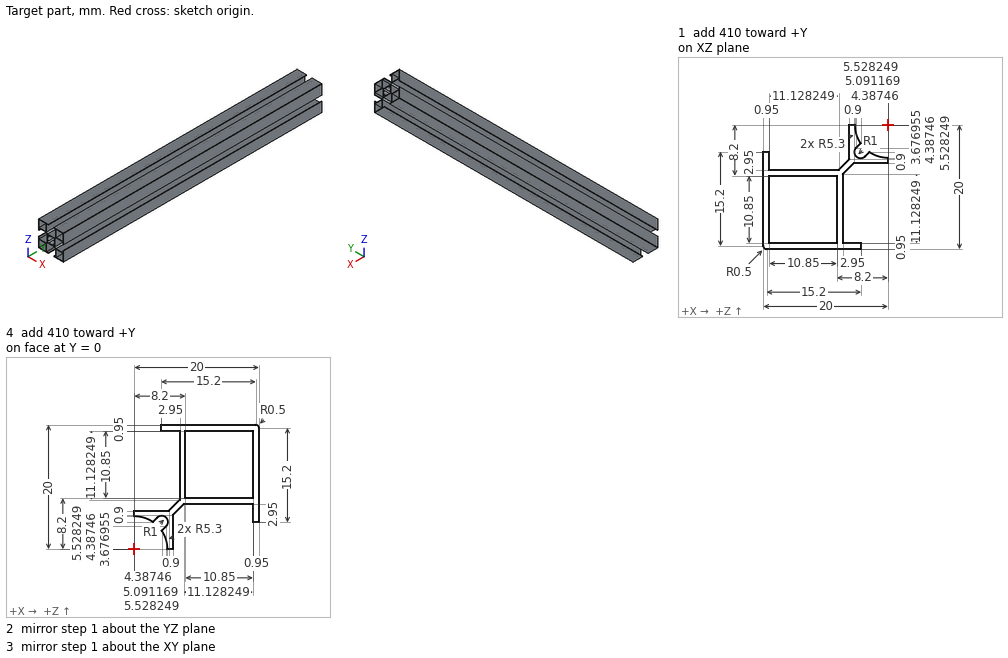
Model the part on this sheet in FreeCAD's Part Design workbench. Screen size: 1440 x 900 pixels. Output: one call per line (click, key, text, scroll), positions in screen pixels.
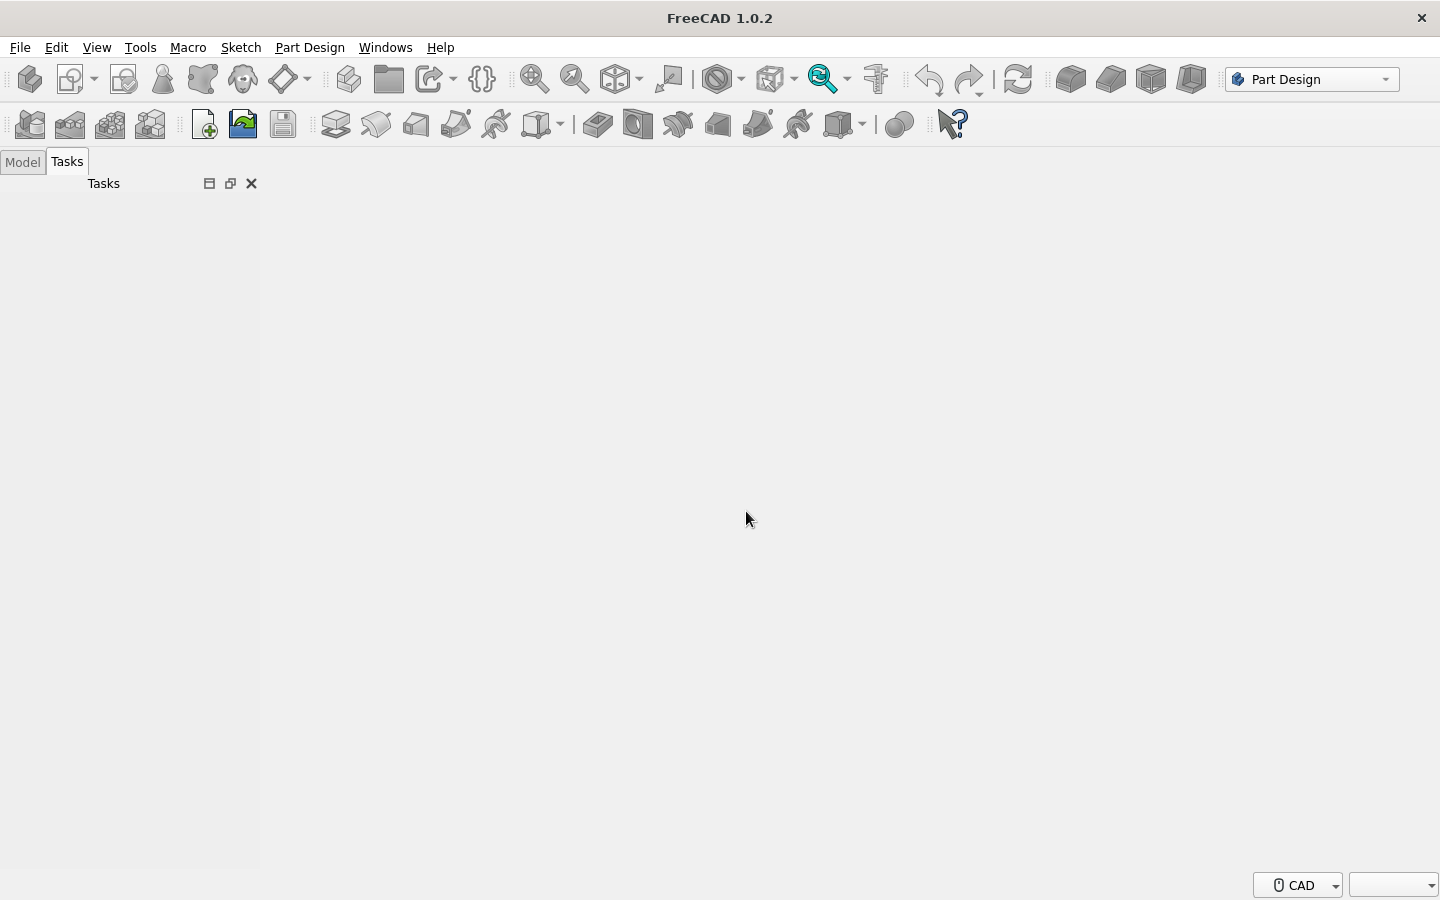
click(204, 124)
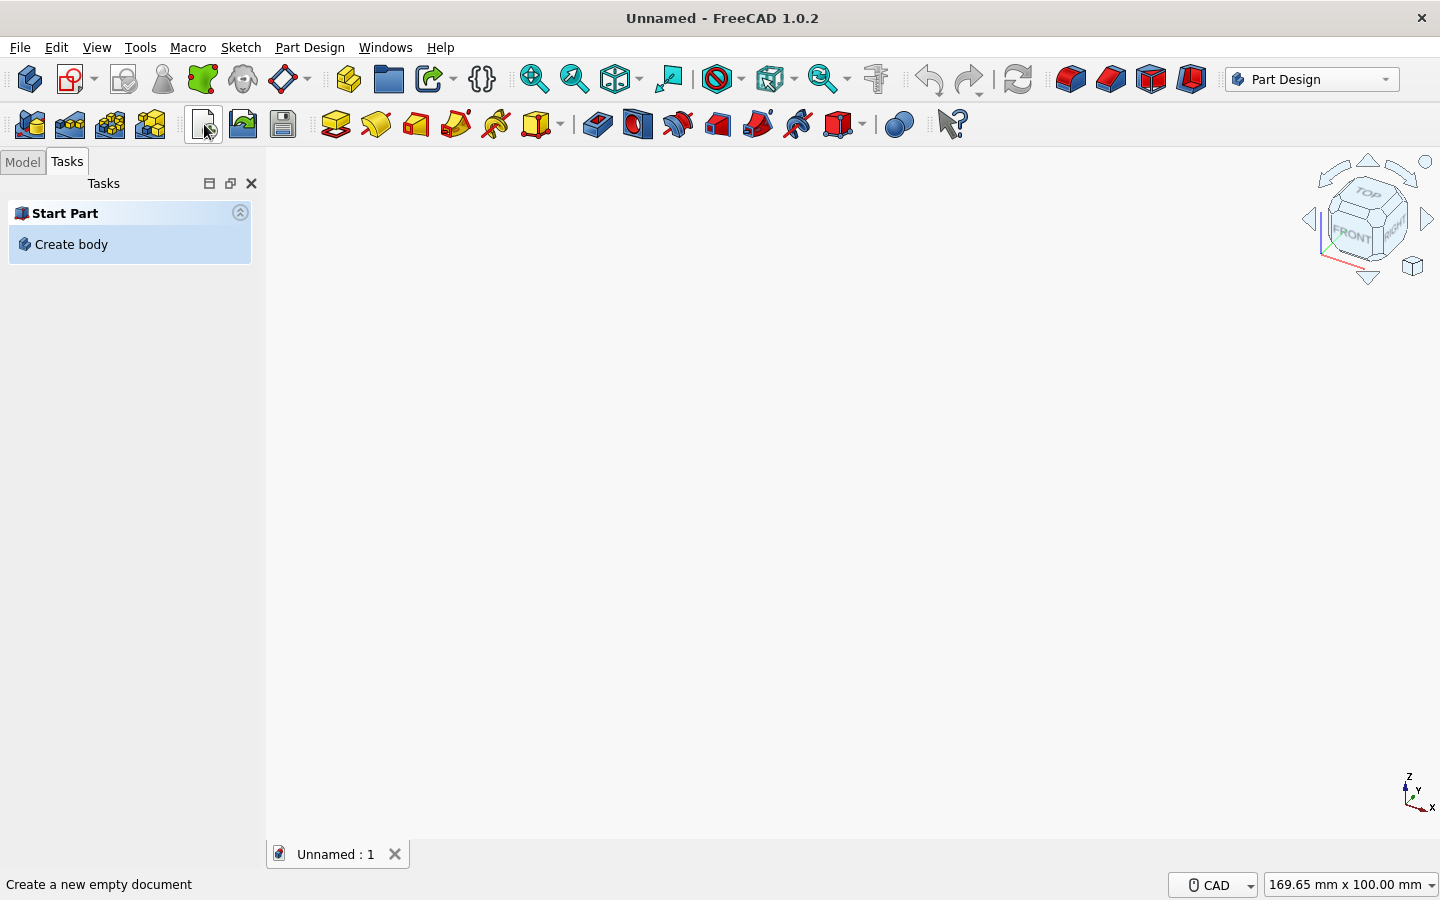
click(70, 80)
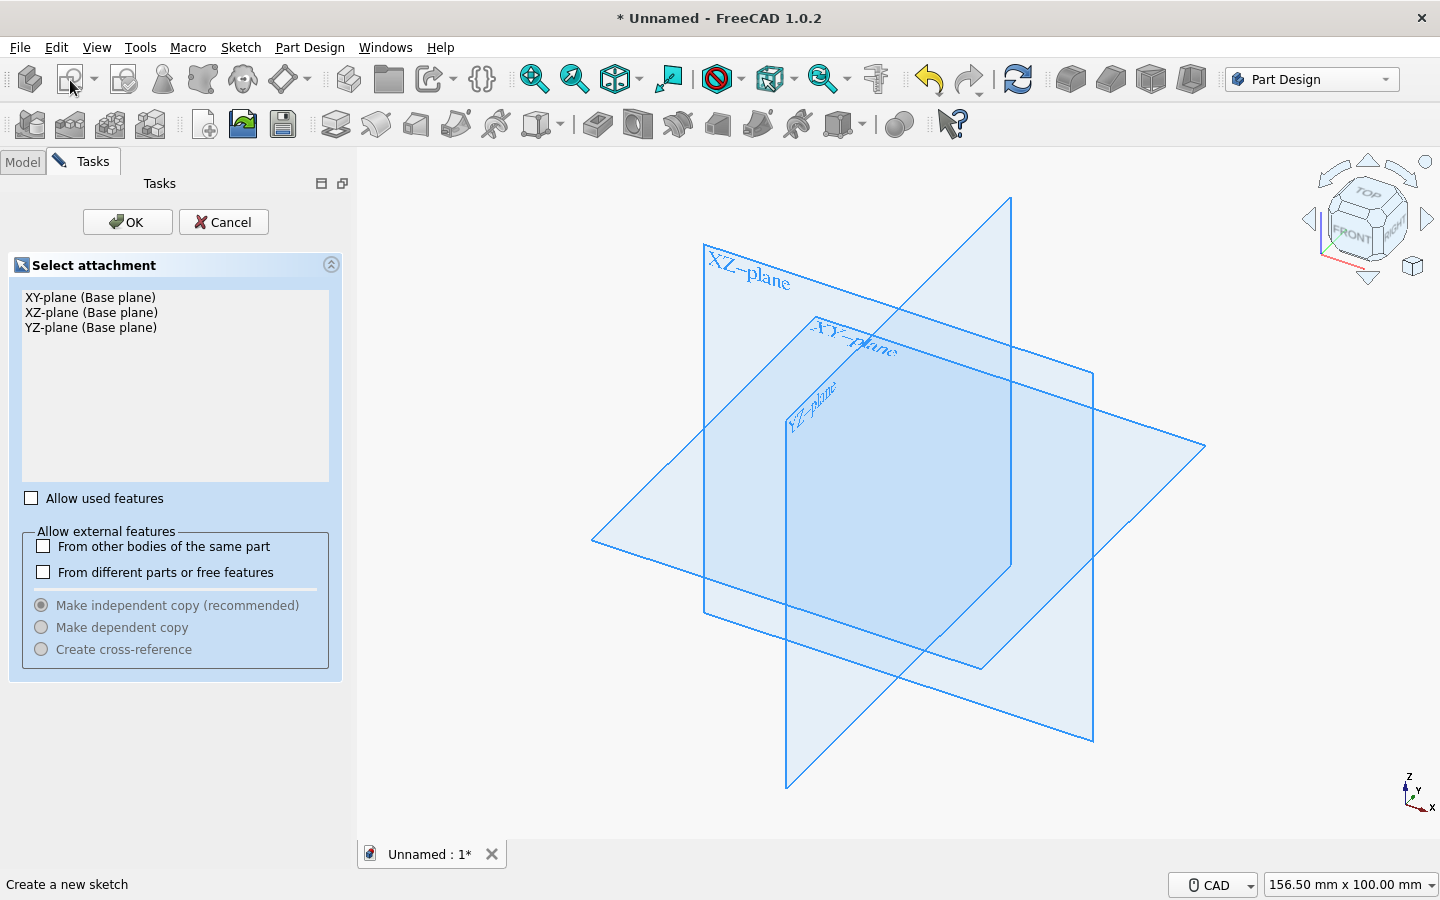
click(82, 312)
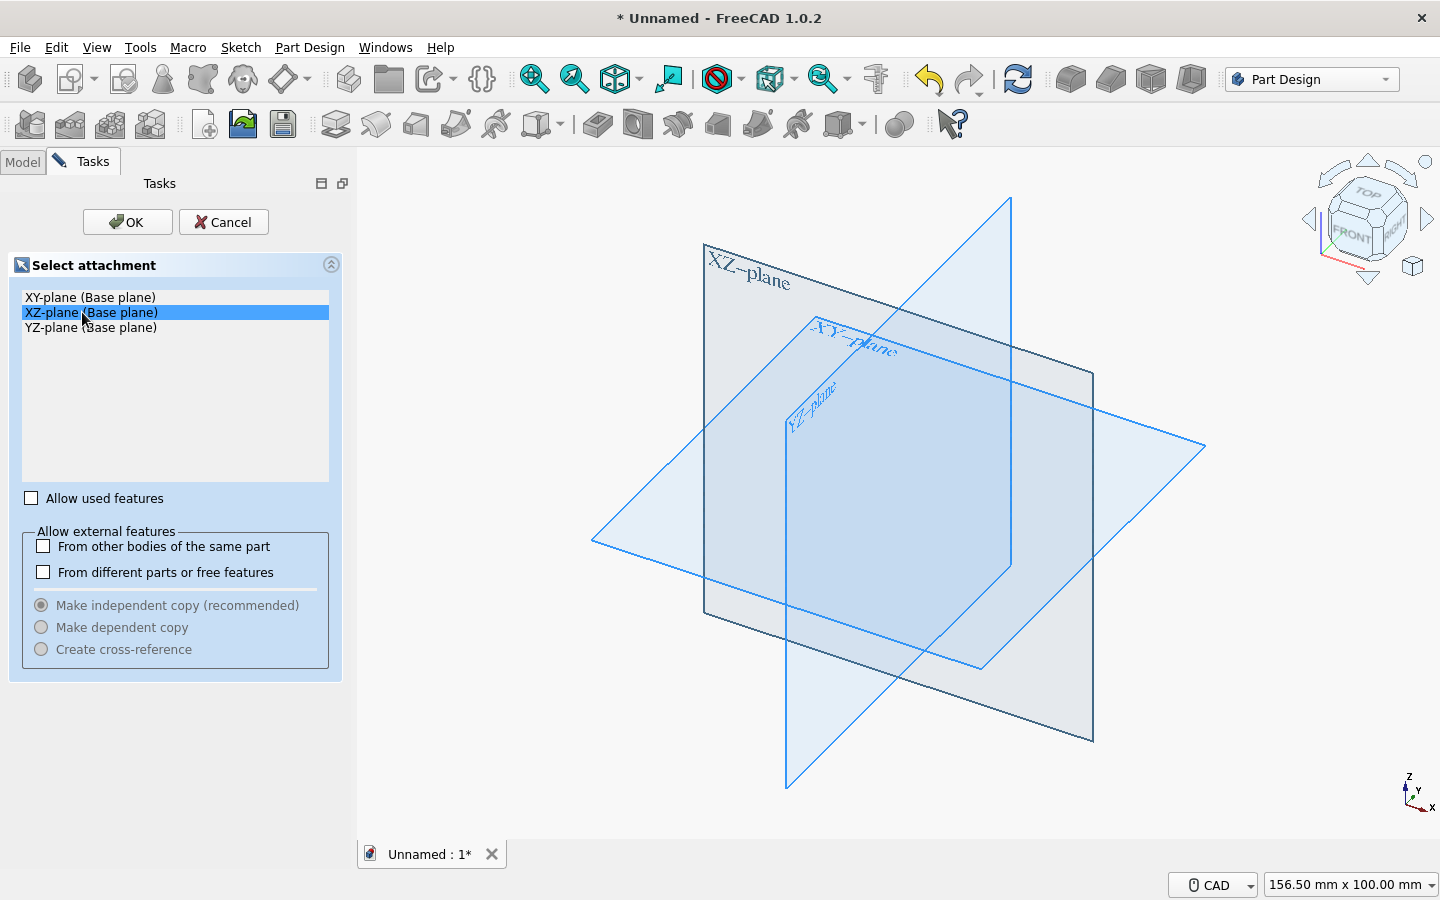
click(128, 222)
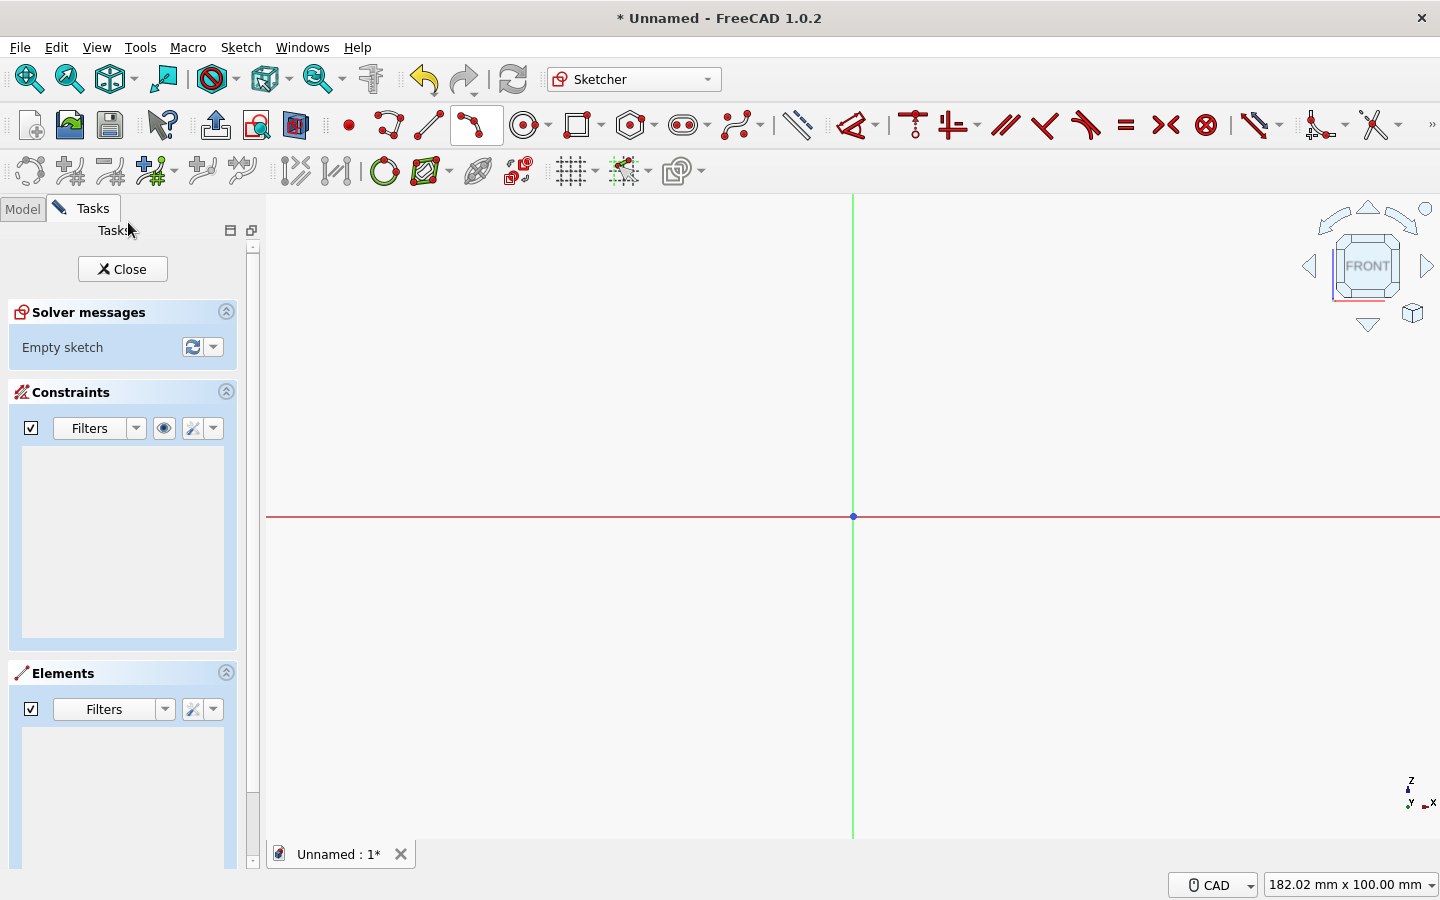
scroll(790, 609, up, 6)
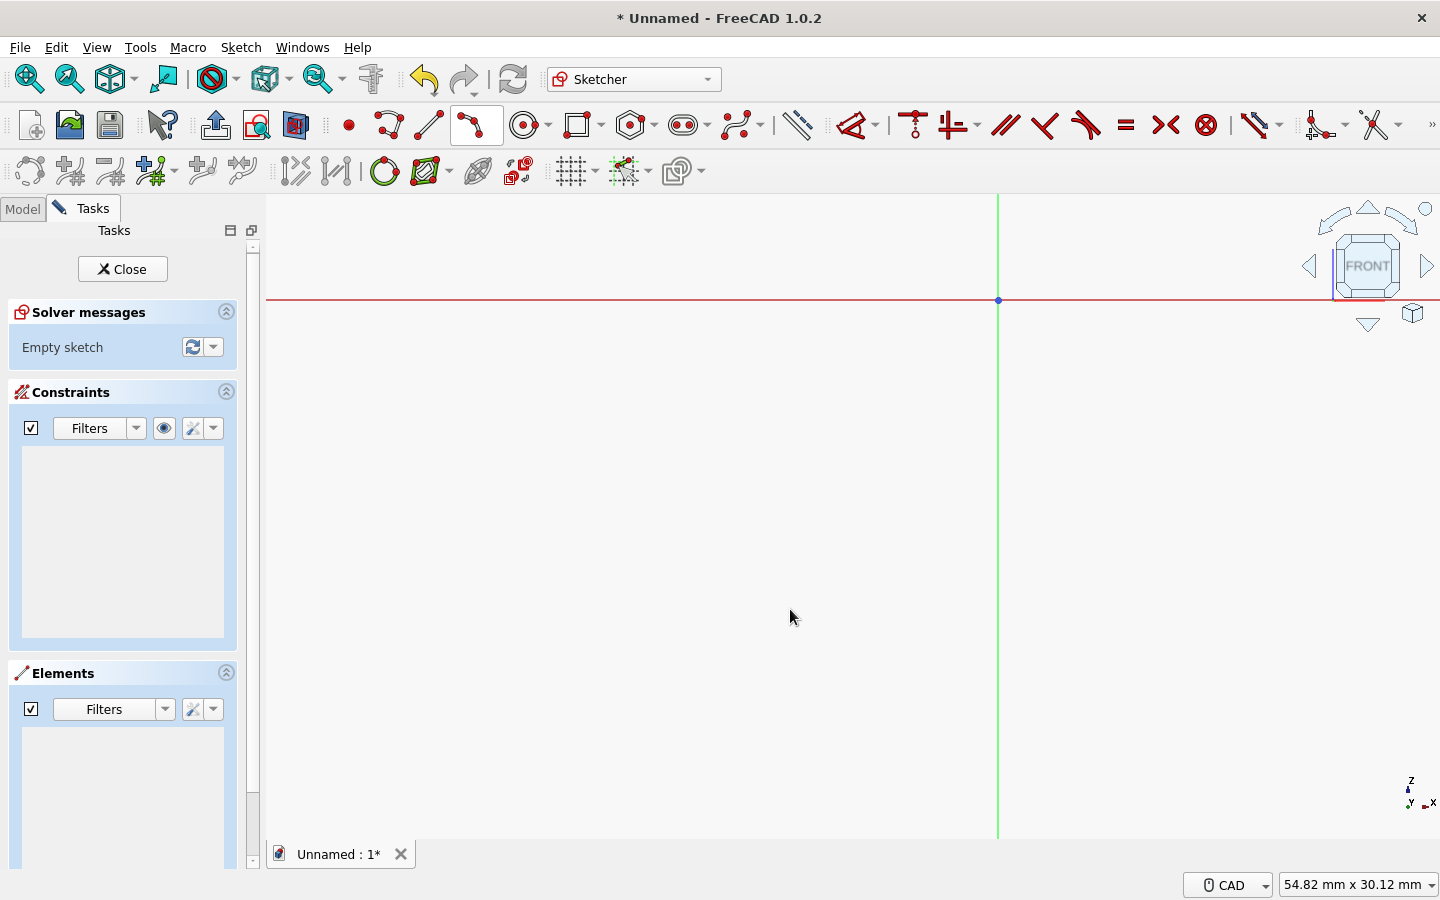
click(390, 126)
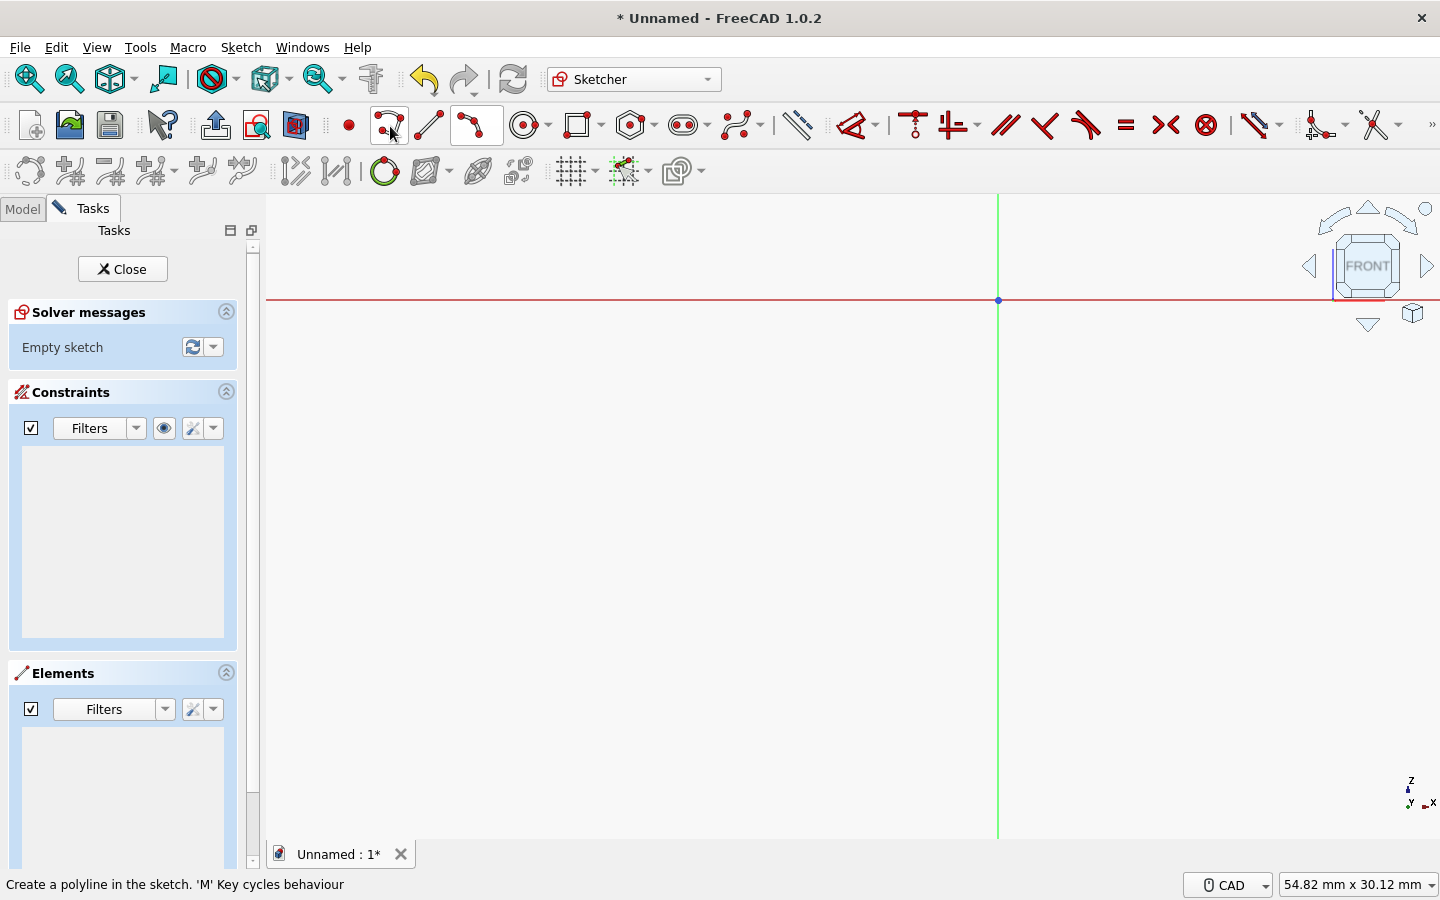
click(570, 718)
click(570, 392)
click(590, 392)
click(590, 456)
click(828, 456)
click(865, 419)
click(865, 300)
click(885, 309)
right_click(885, 309)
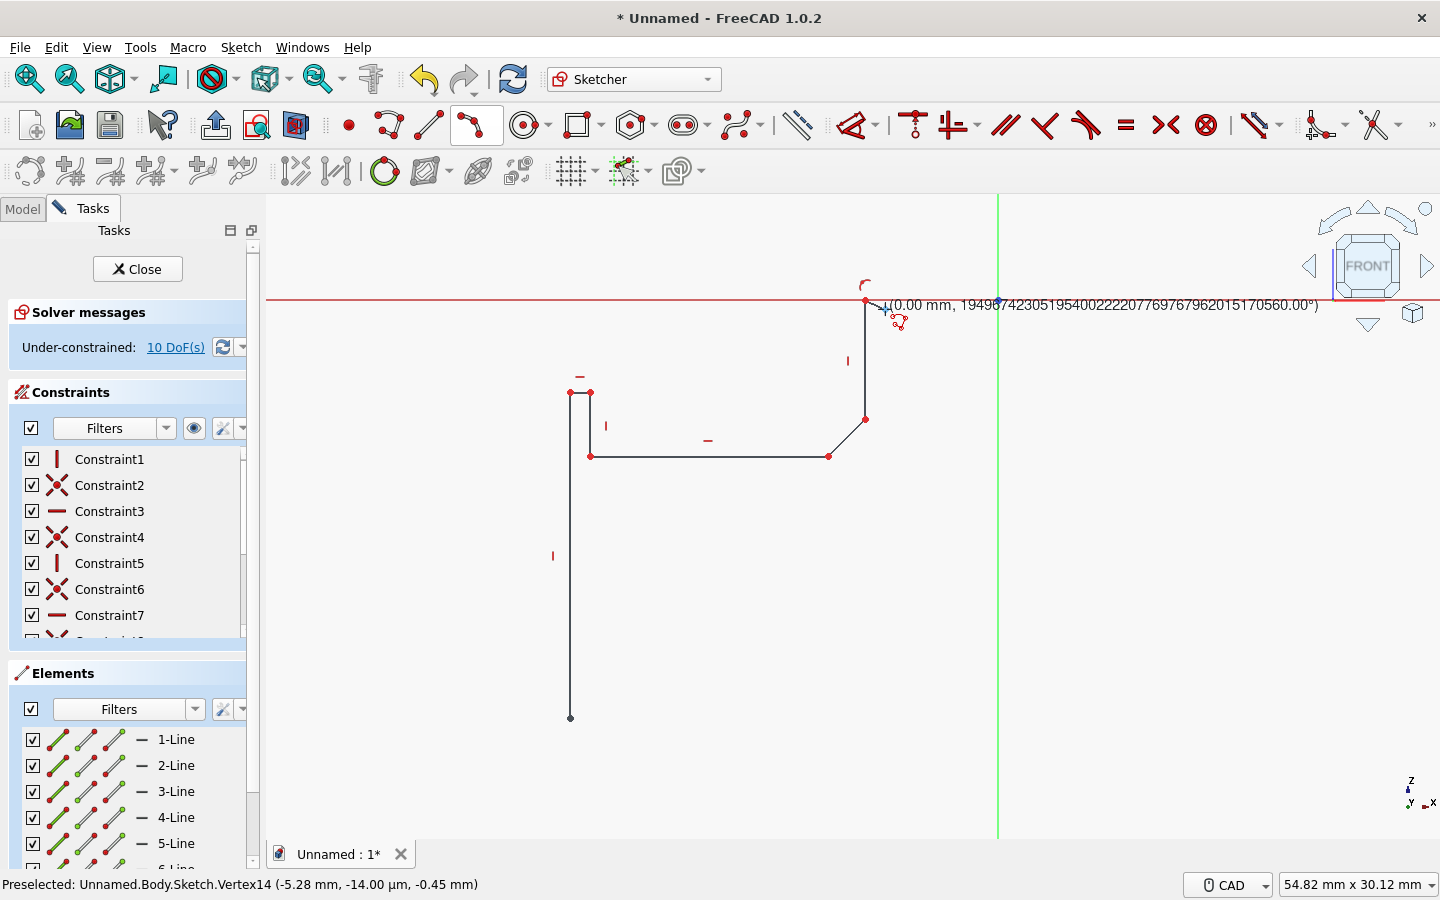
click(430, 126)